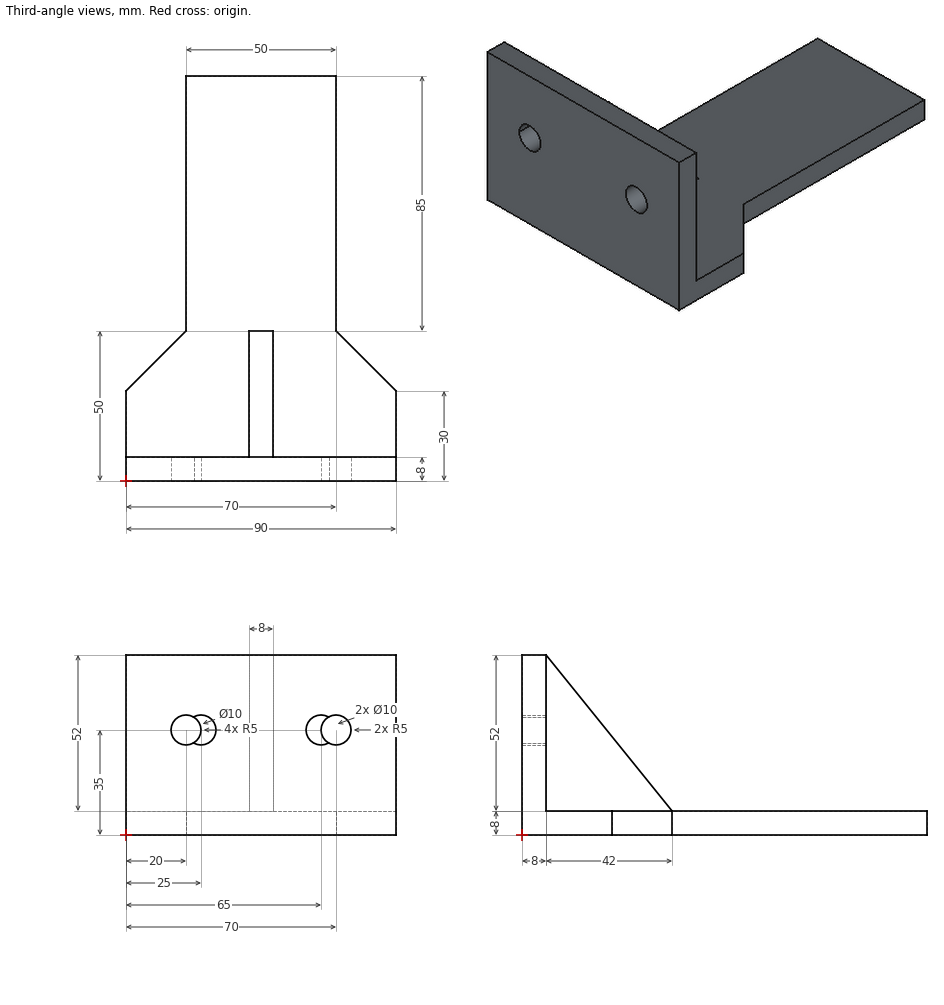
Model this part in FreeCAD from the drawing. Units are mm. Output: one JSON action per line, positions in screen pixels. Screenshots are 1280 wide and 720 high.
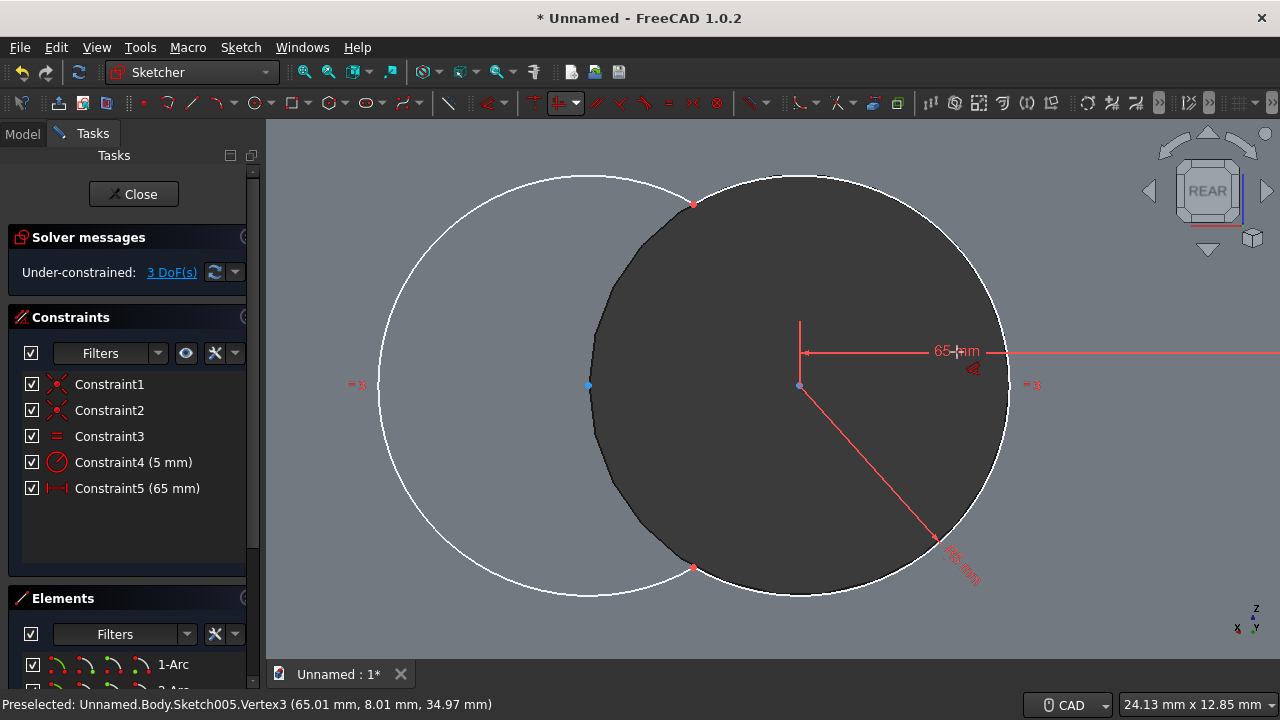
{"action": "left_click", "coordinate": [800, 386]}
{"action": "left_click", "coordinate": [766, 508]}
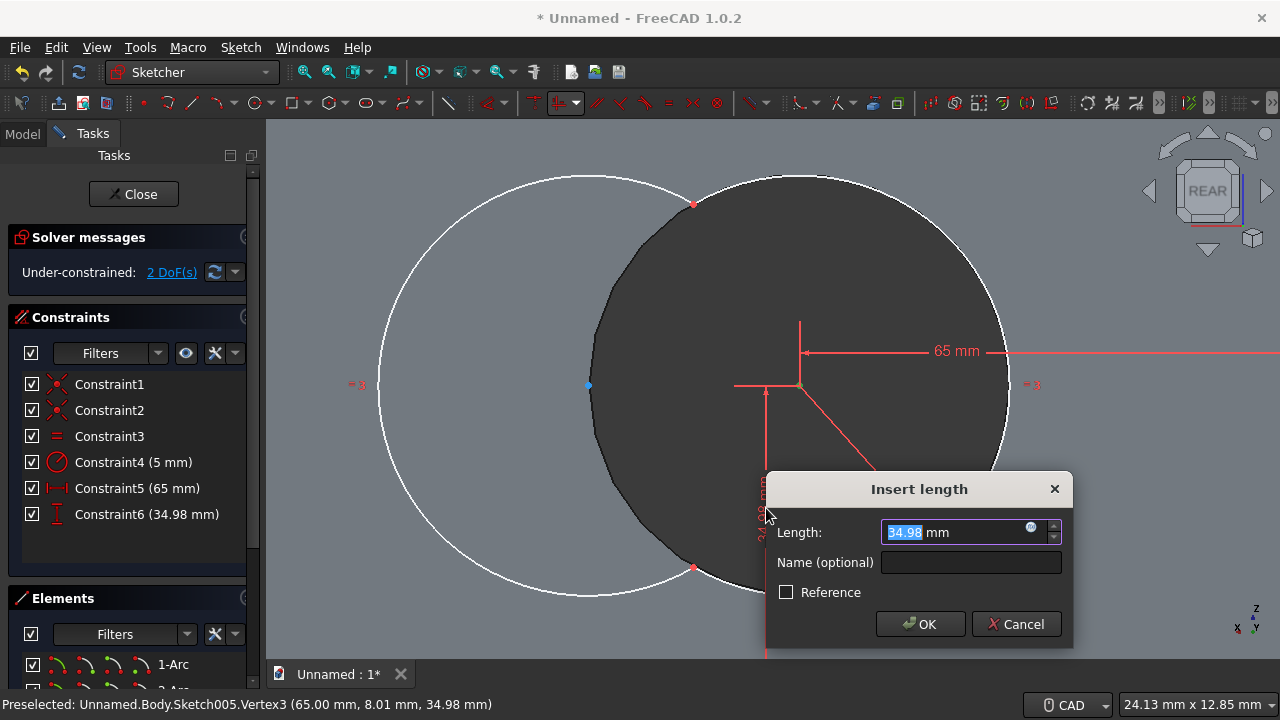
{"action": "type", "text": "35"}
{"action": "key", "text": "Return"}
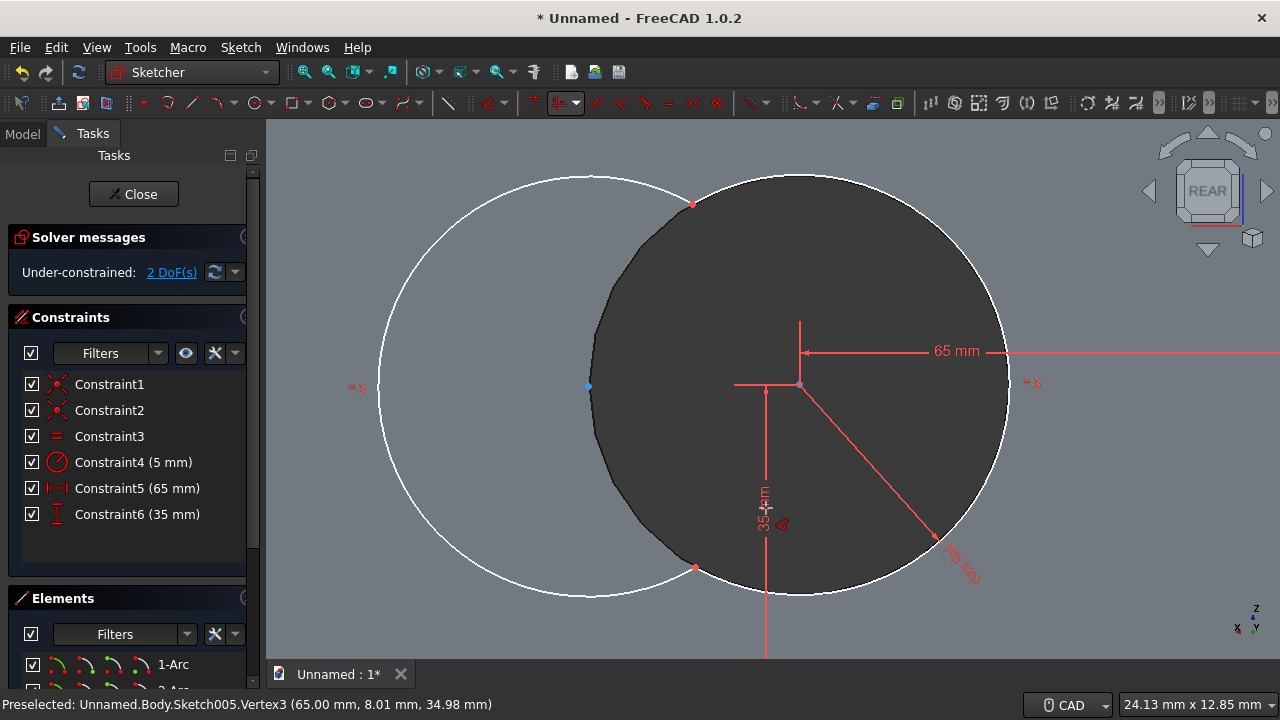
{"action": "left_click", "coordinate": [588, 387]}
{"action": "left_click", "coordinate": [852, 353]}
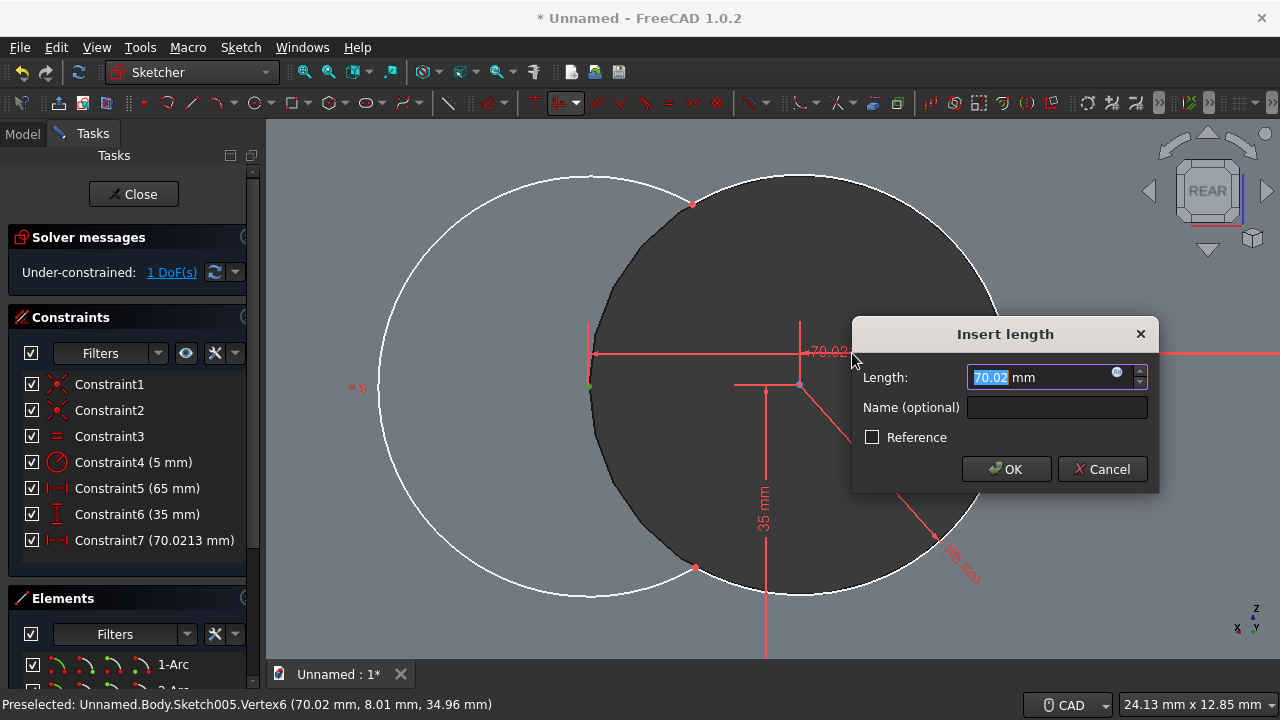
{"action": "type", "text": "70"}
{"action": "key", "text": "Return"}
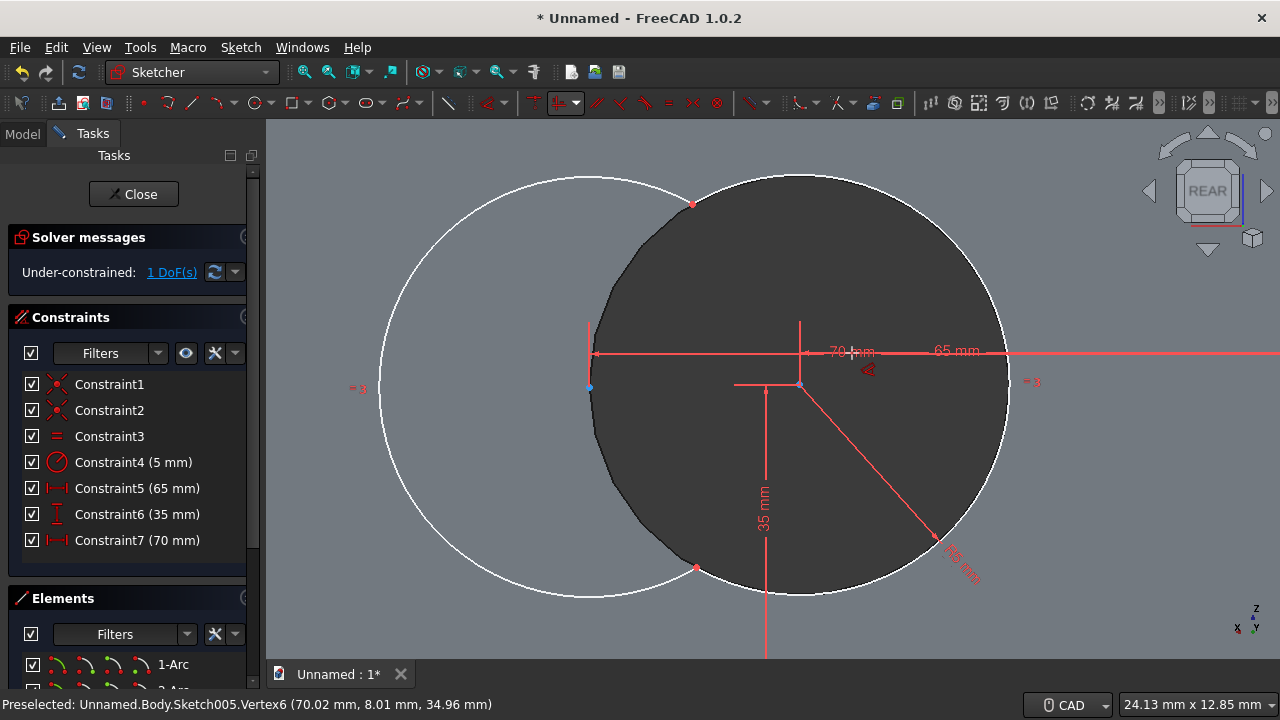
{"action": "left_click", "coordinate": [589, 387]}
{"action": "left_click", "coordinate": [555, 509]}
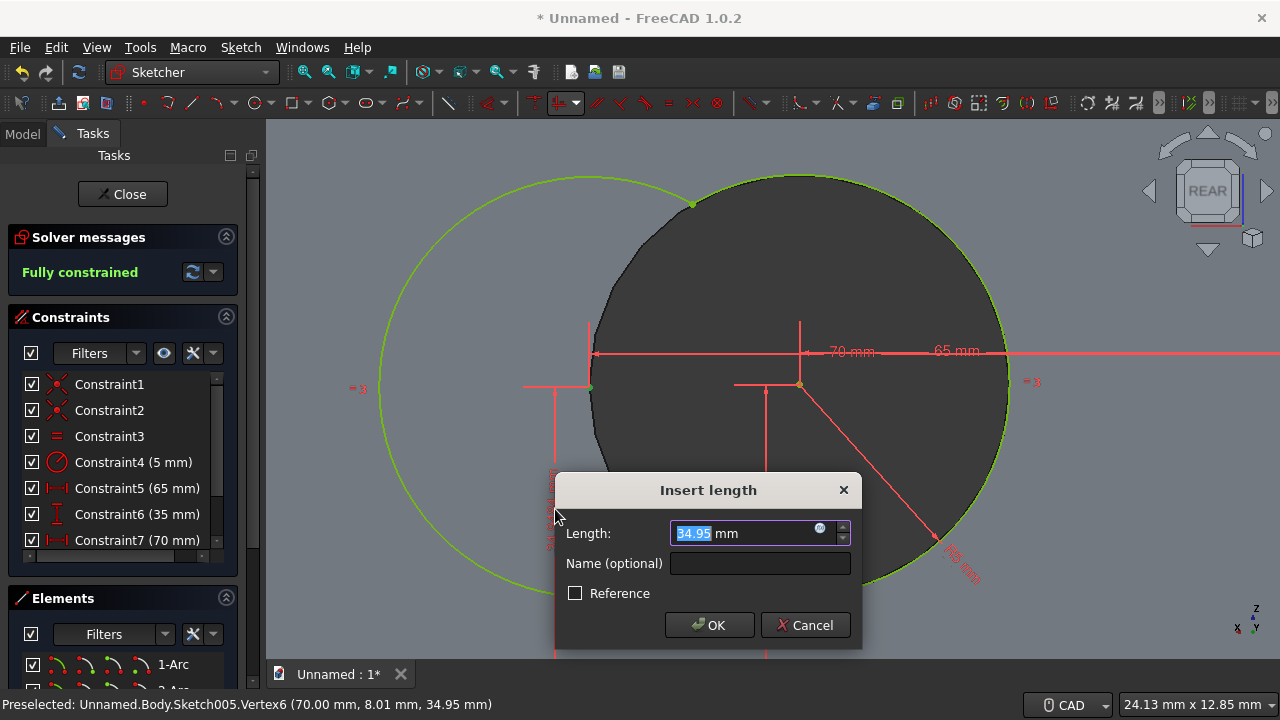
{"action": "type", "text": "35"}
{"action": "key", "text": "Return"}
{"action": "key", "text": "Escape"}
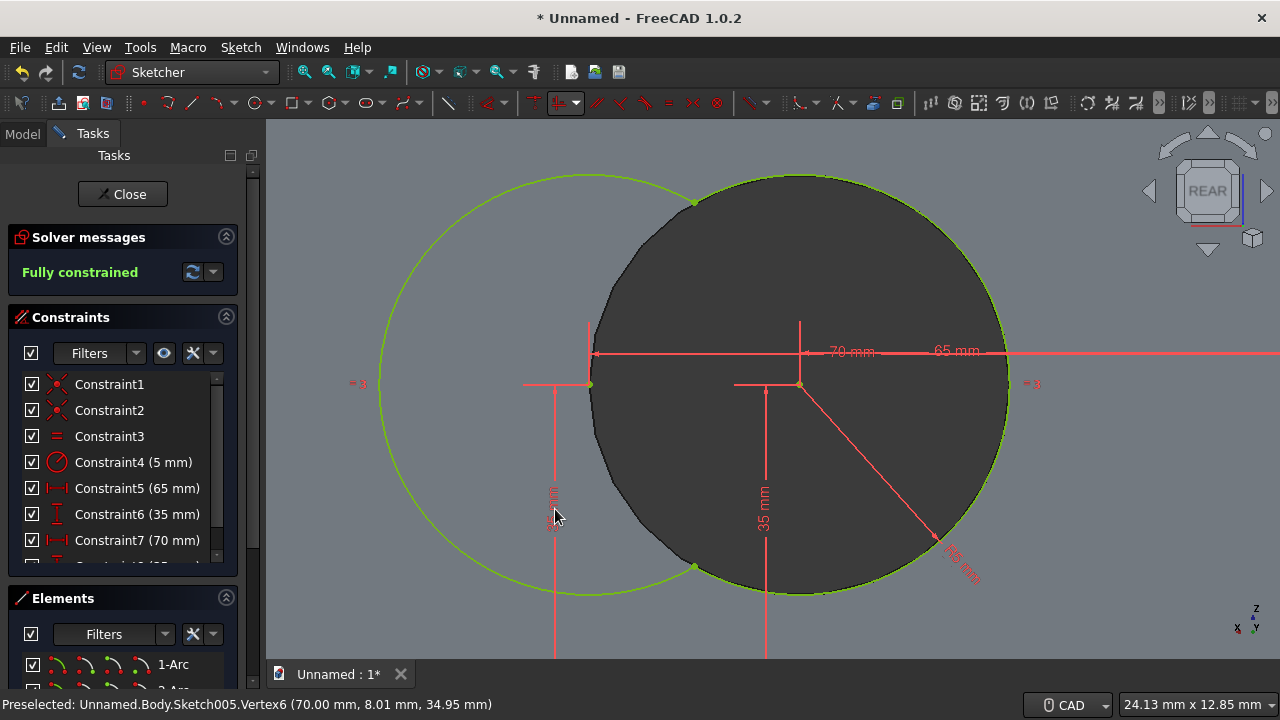
{"action": "left_click", "coordinate": [123, 194]}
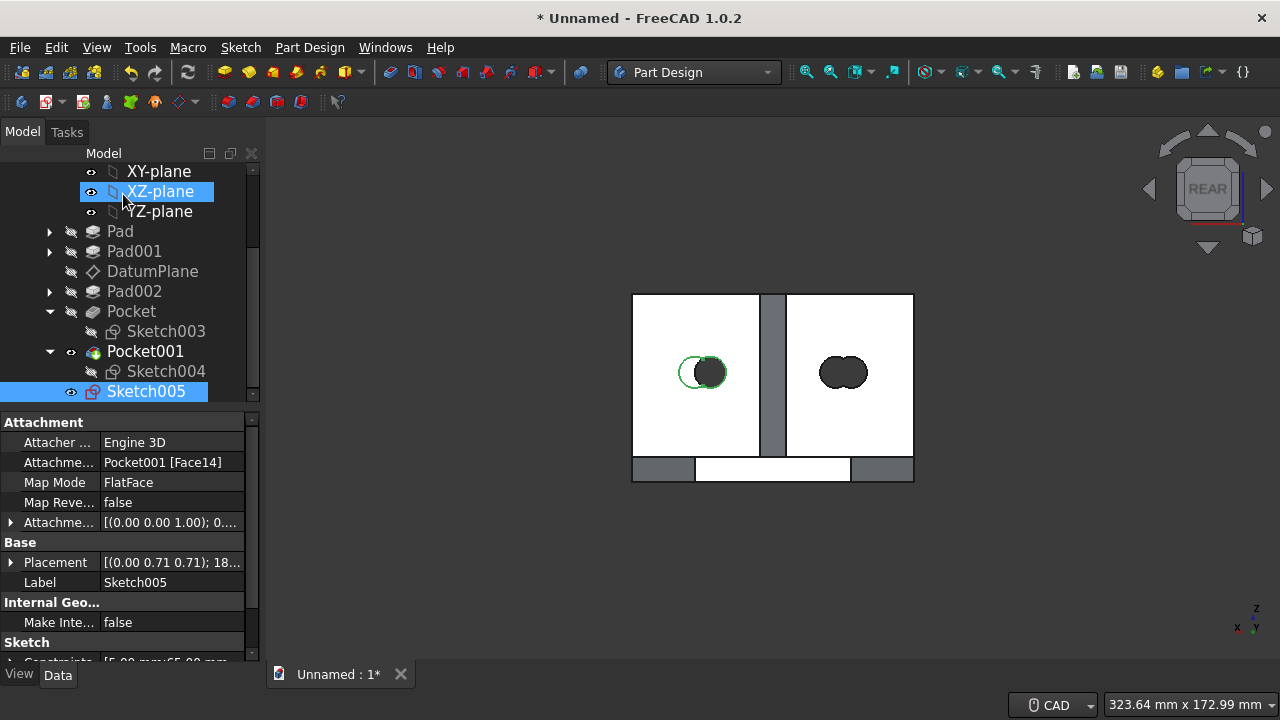
{"action": "left_click", "coordinate": [392, 72]}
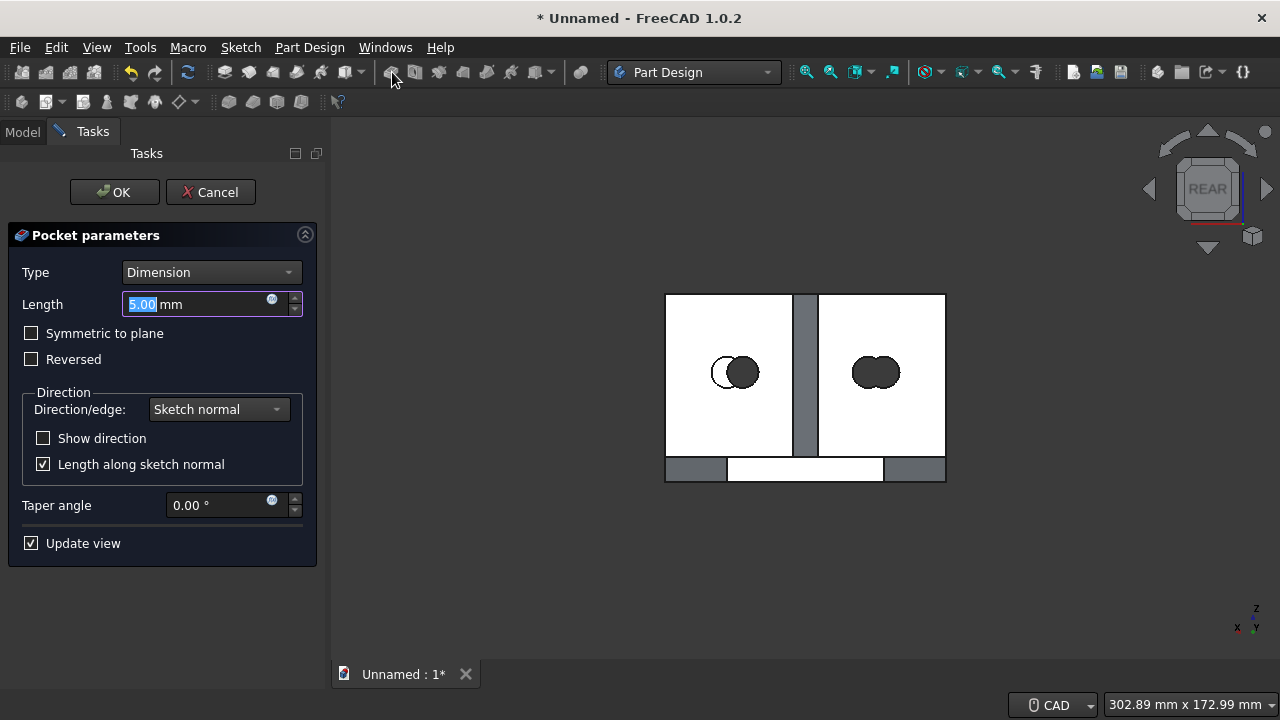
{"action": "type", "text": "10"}
{"action": "key", "text": "Tab"}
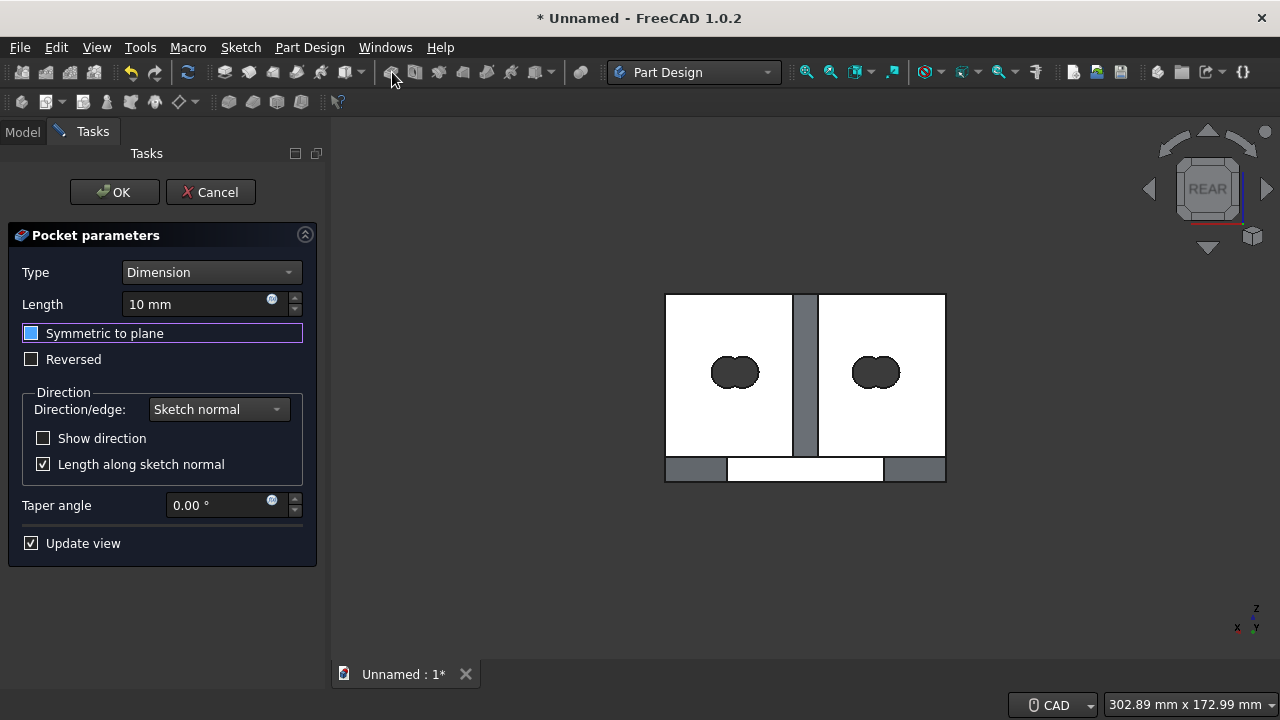
{"action": "left_click", "coordinate": [115, 192]}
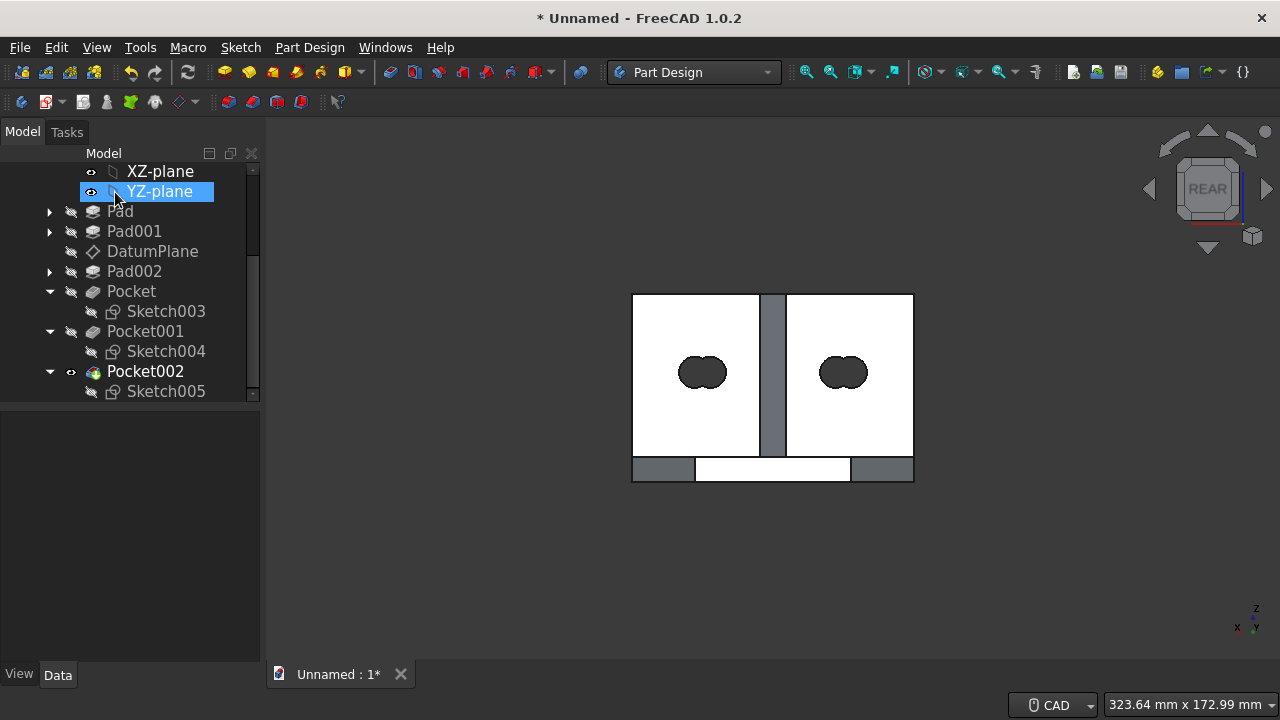
{"action": "left_click", "coordinate": [808, 72]}